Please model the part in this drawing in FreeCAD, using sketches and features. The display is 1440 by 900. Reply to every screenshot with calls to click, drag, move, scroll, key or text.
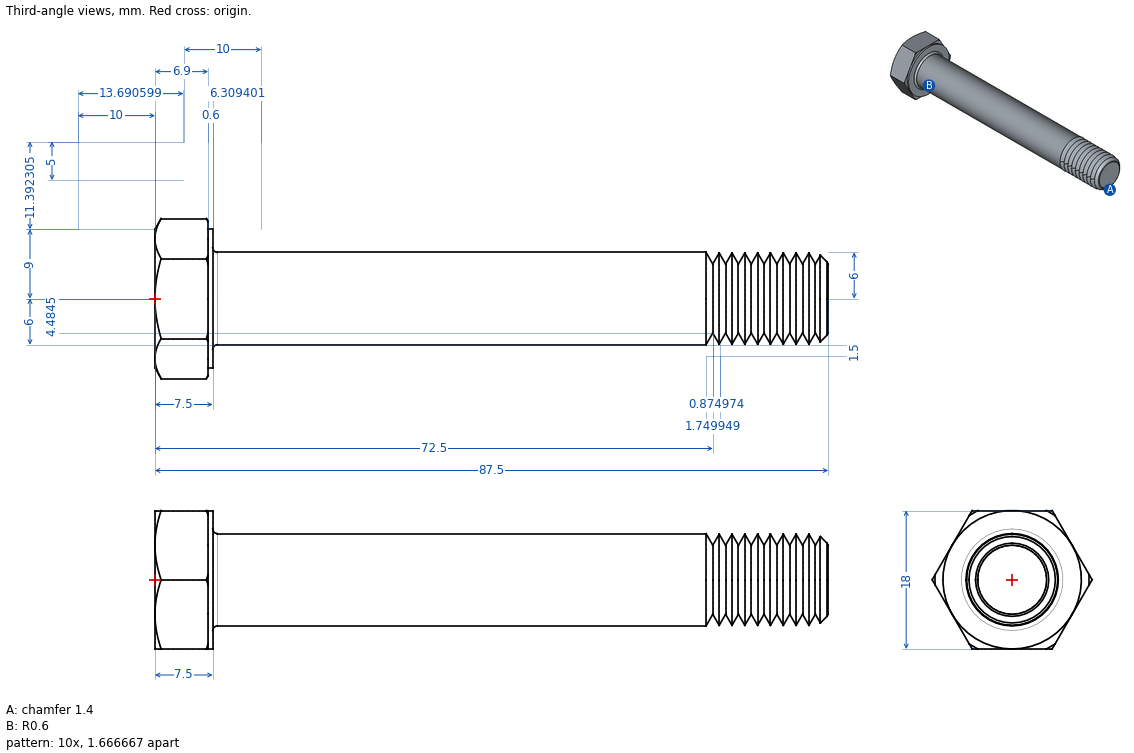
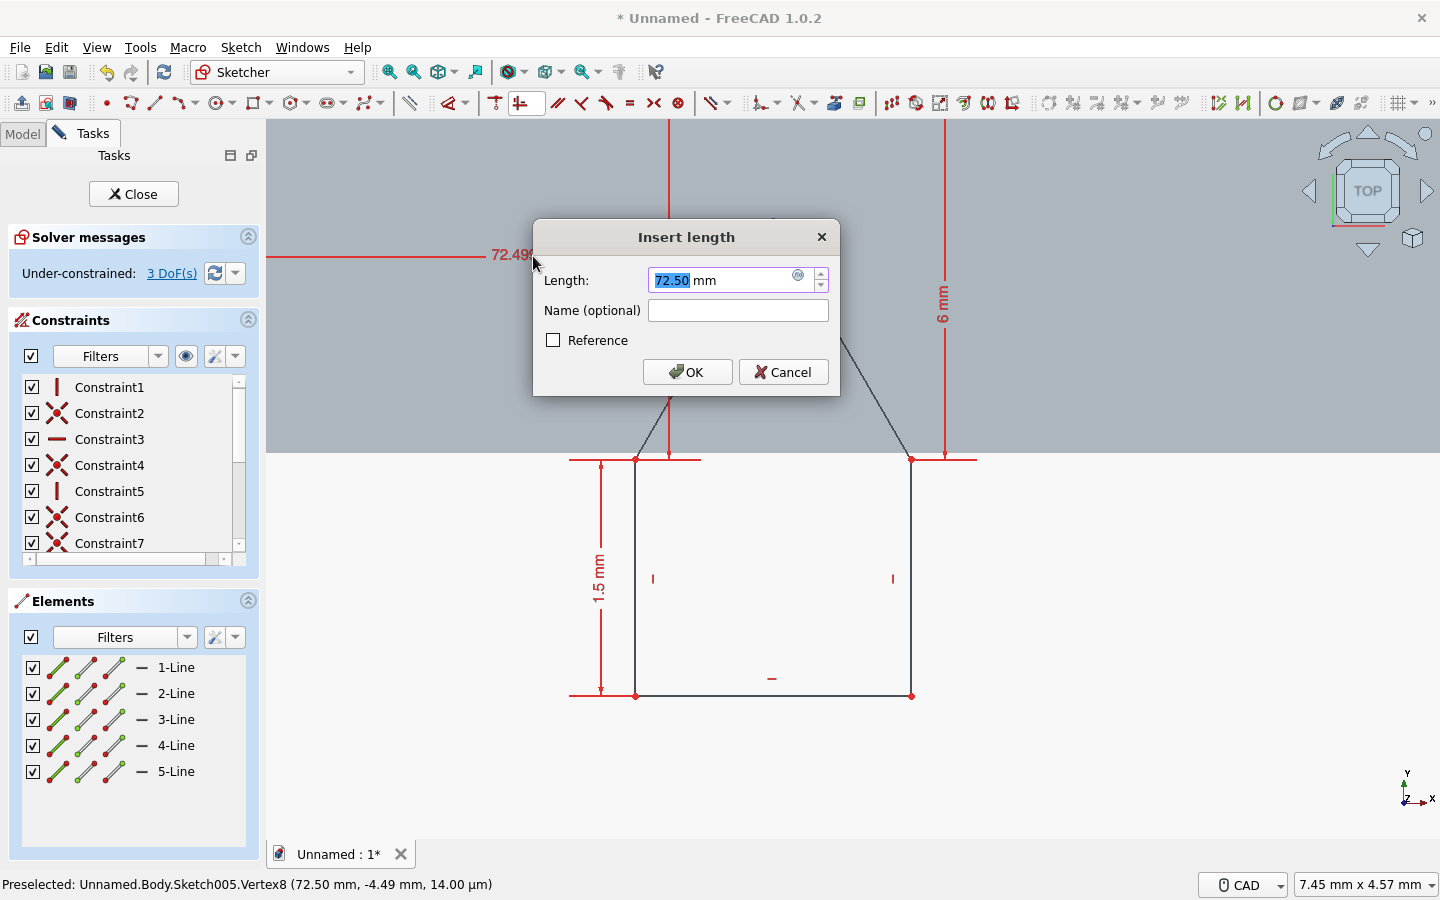
text(72.5)
key(Return)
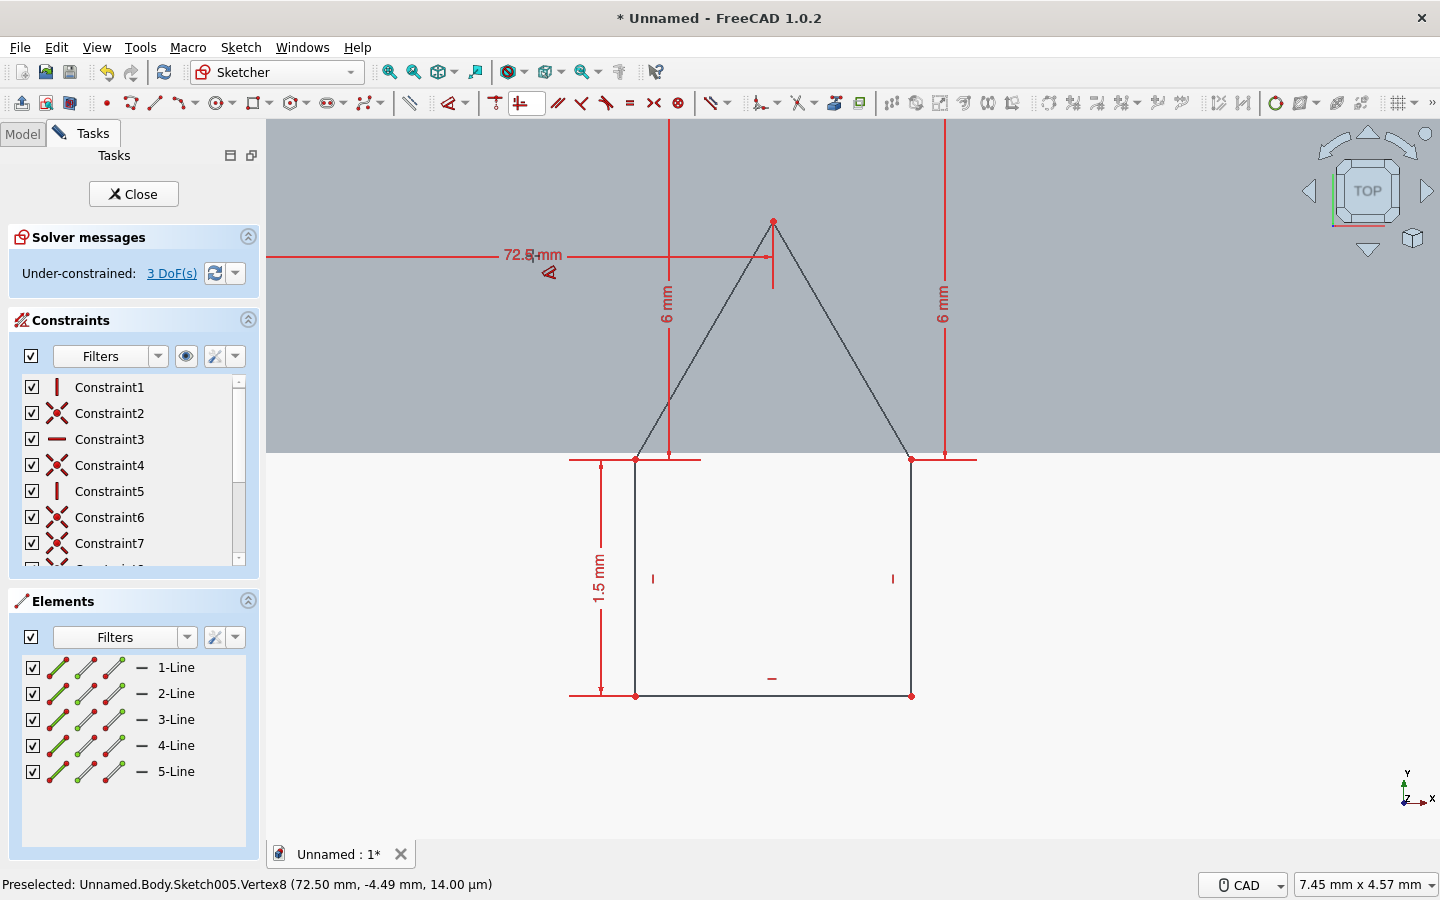
click(773, 222)
click(807, 184)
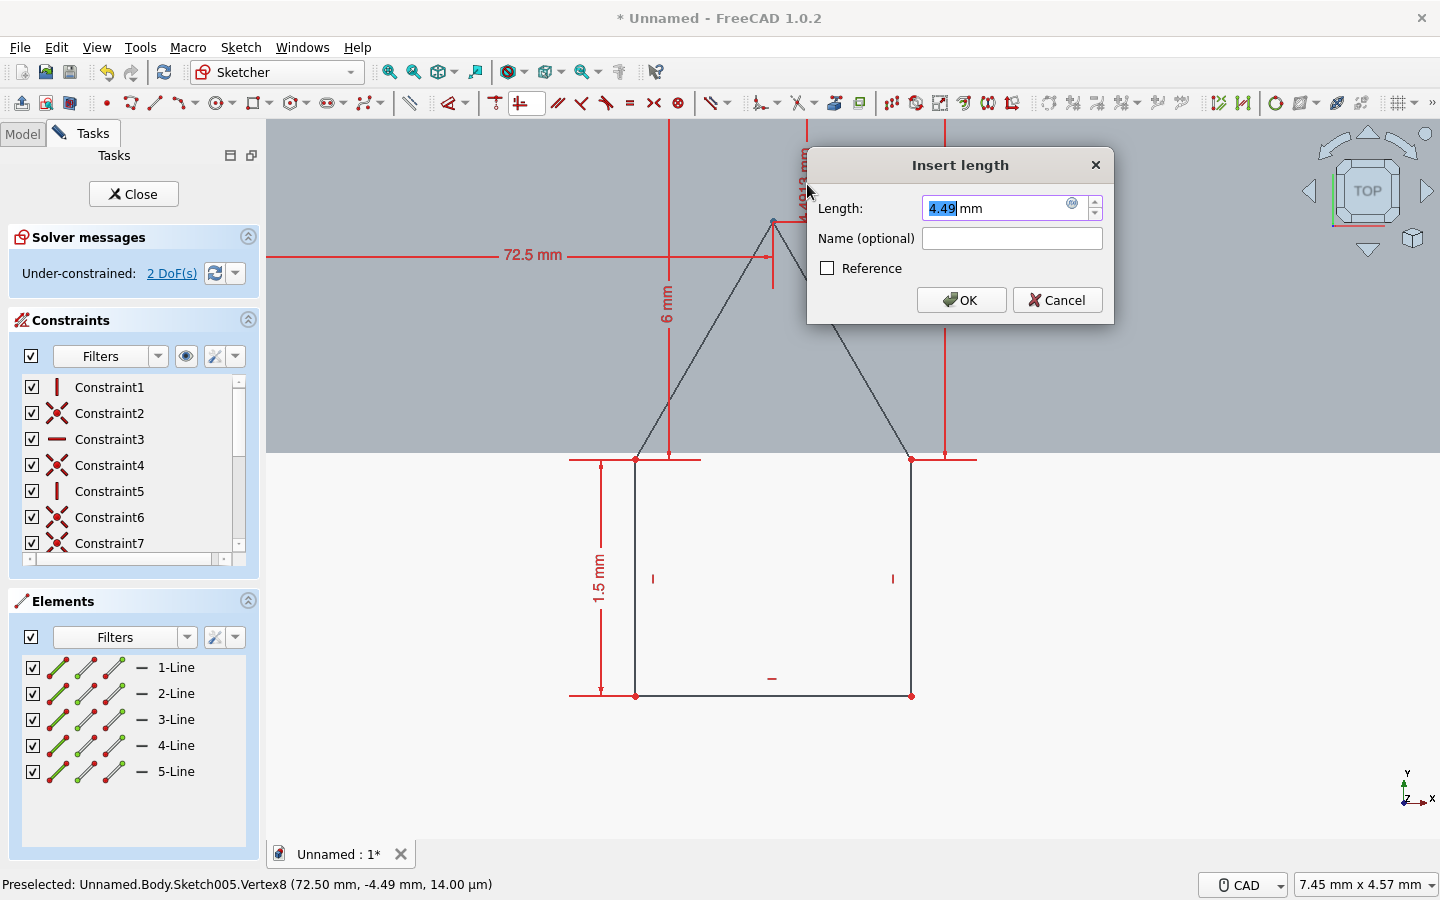
text(4.4845)
key(Return)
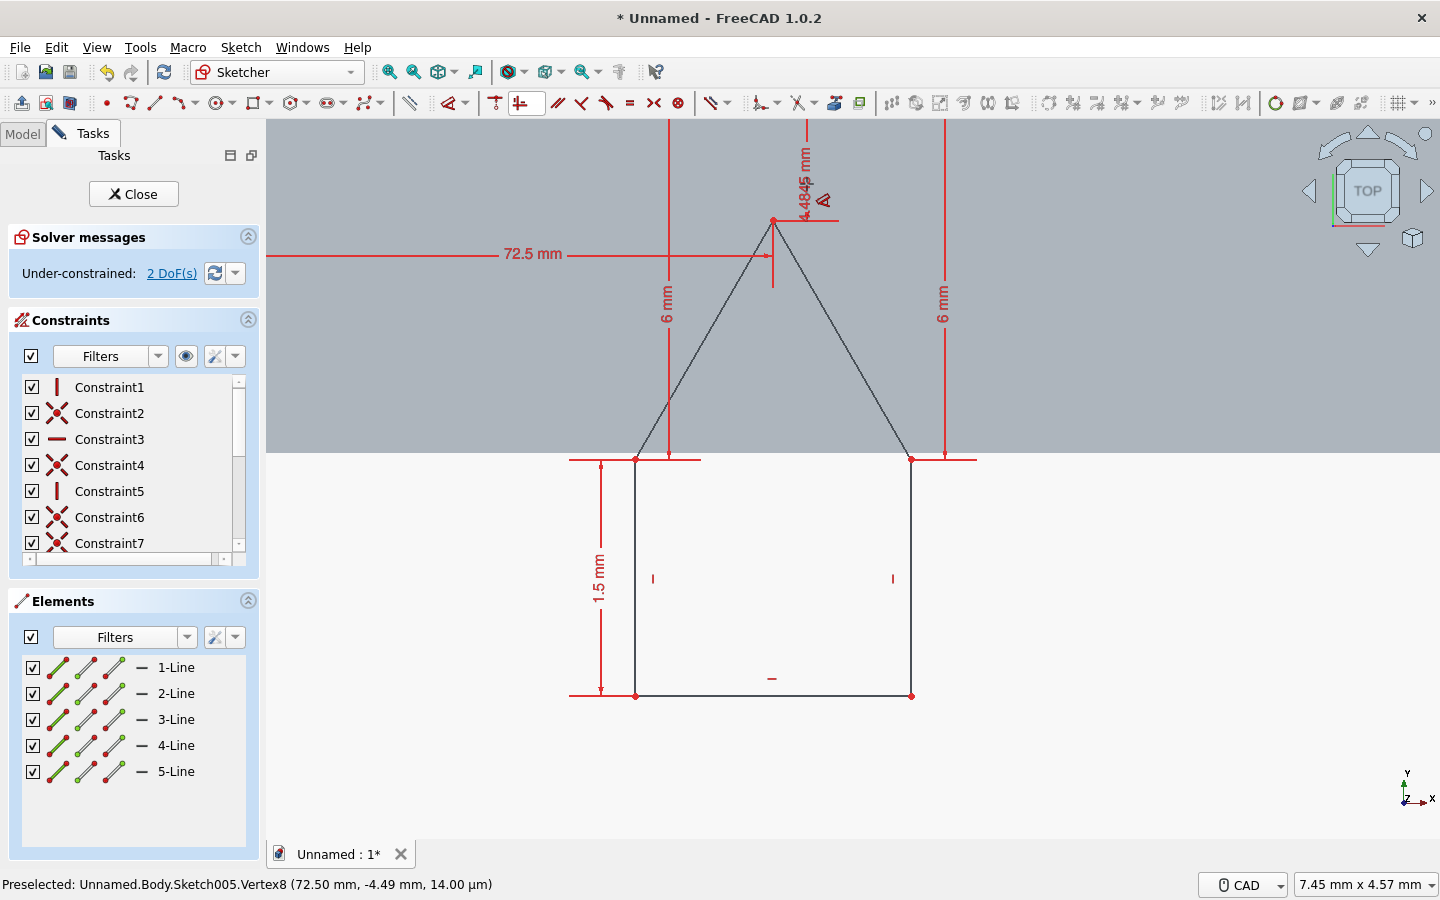
click(718, 696)
click(773, 730)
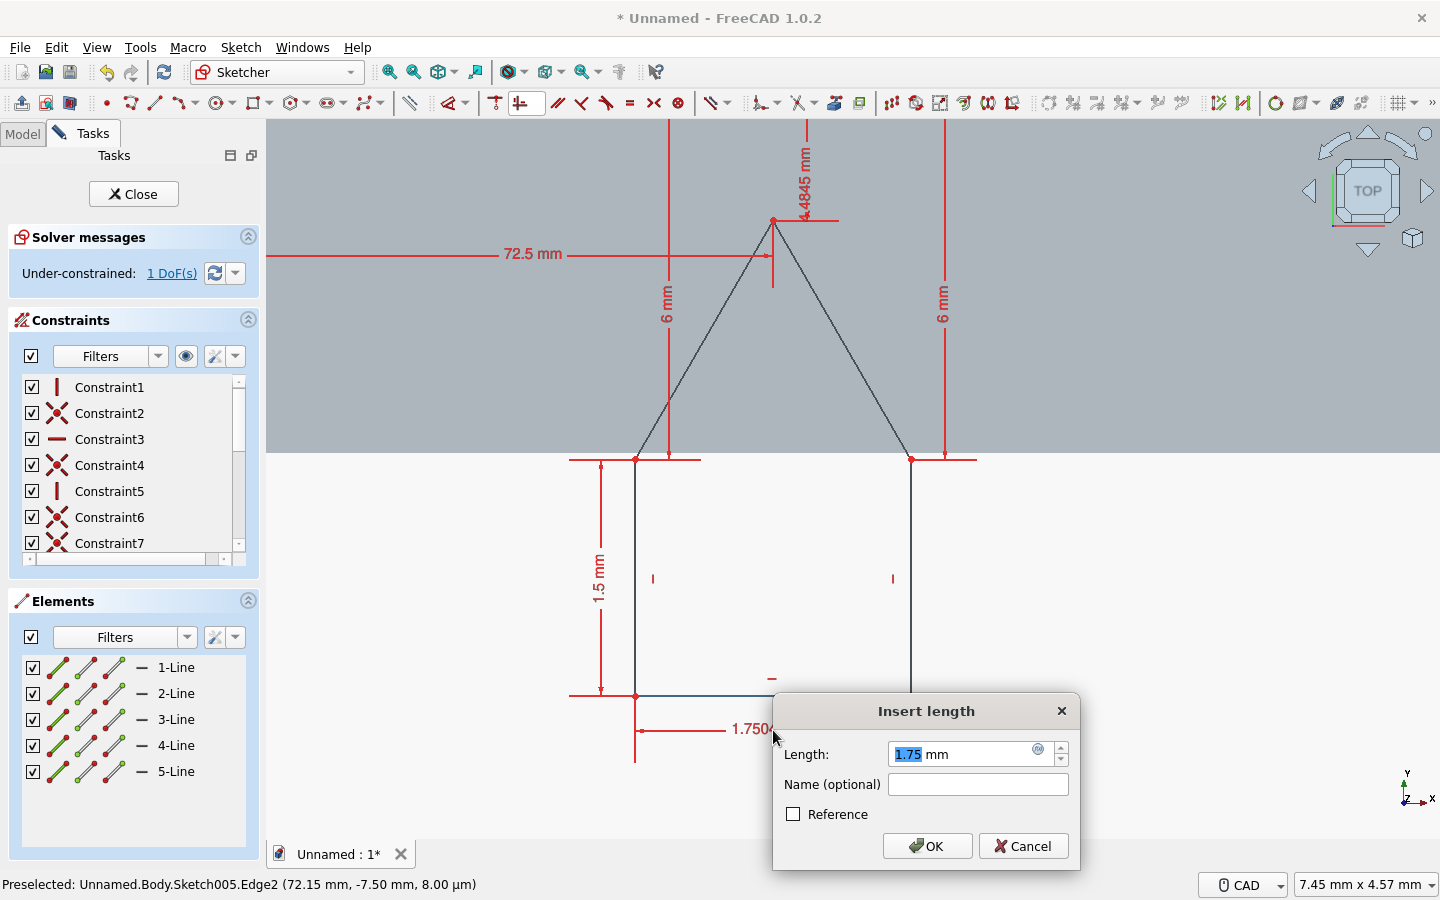
text(1.749949)
key(Return)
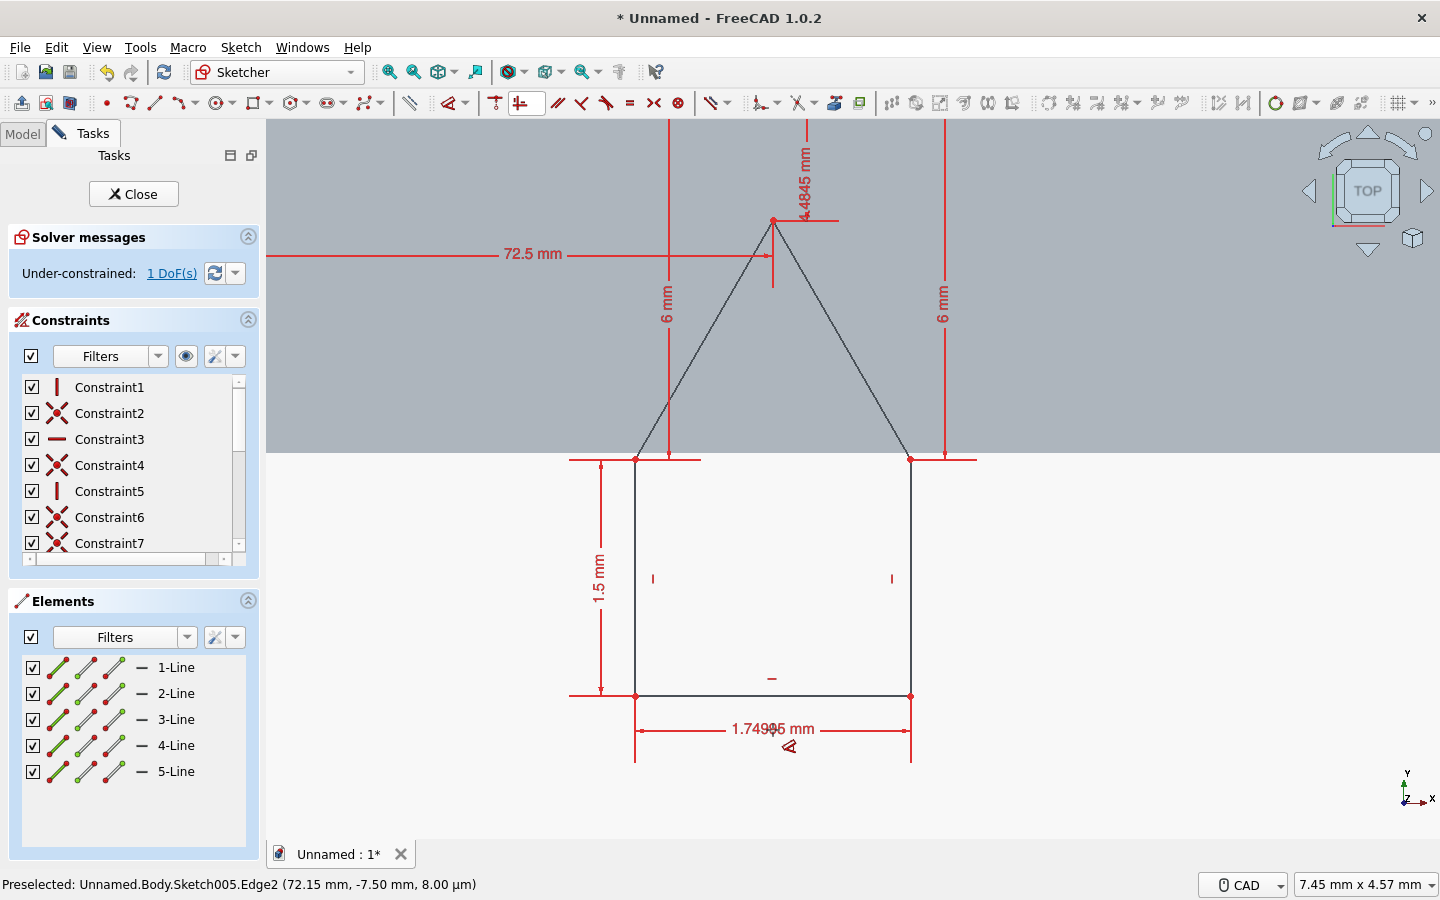
click(870, 388)
click(890, 187)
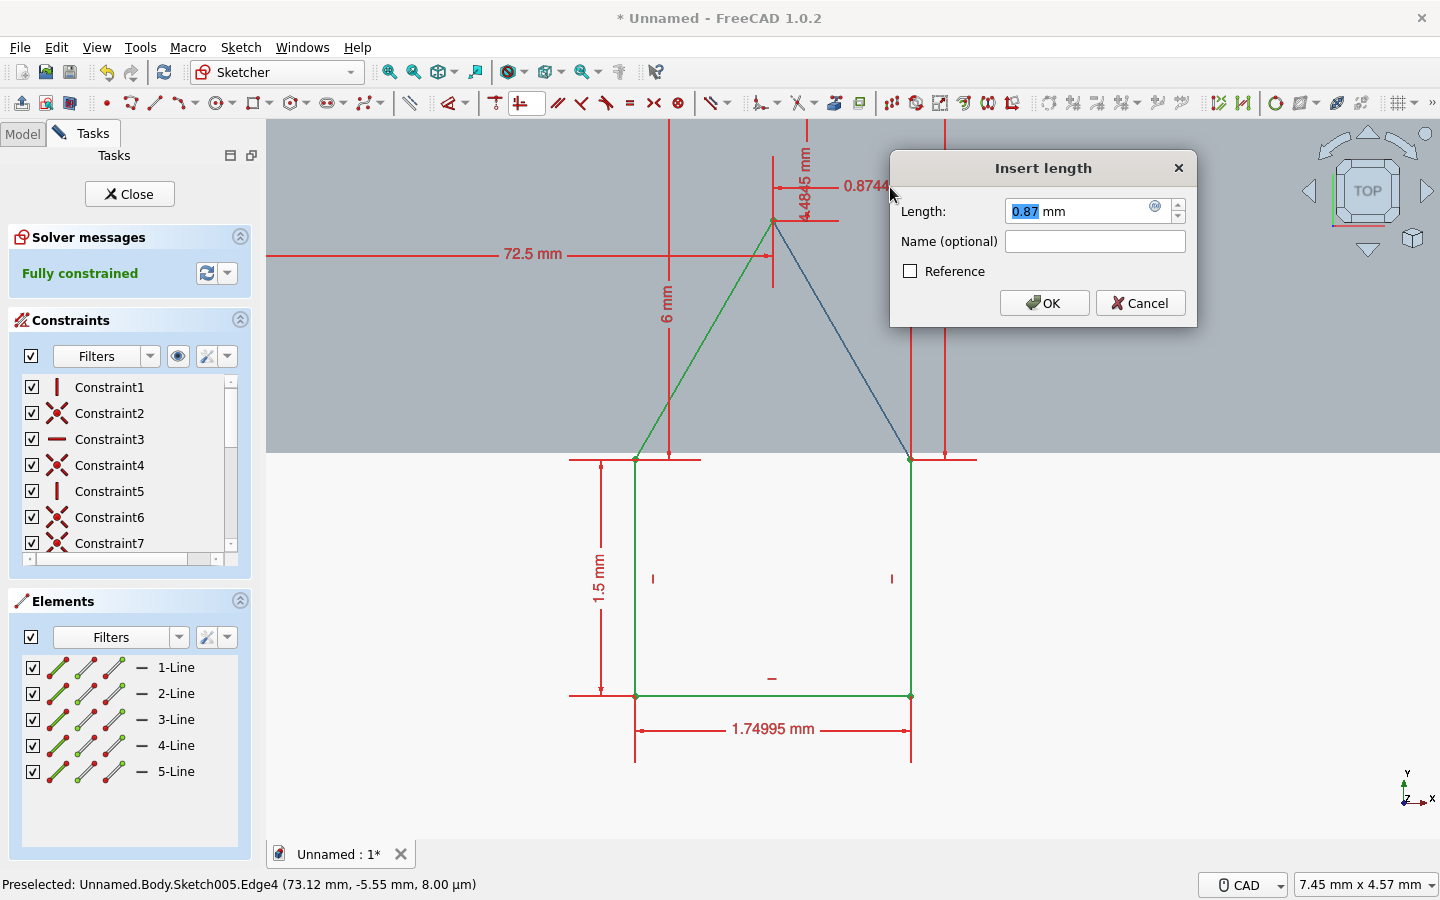
text(0.874974)
key(Return)
key(Escape)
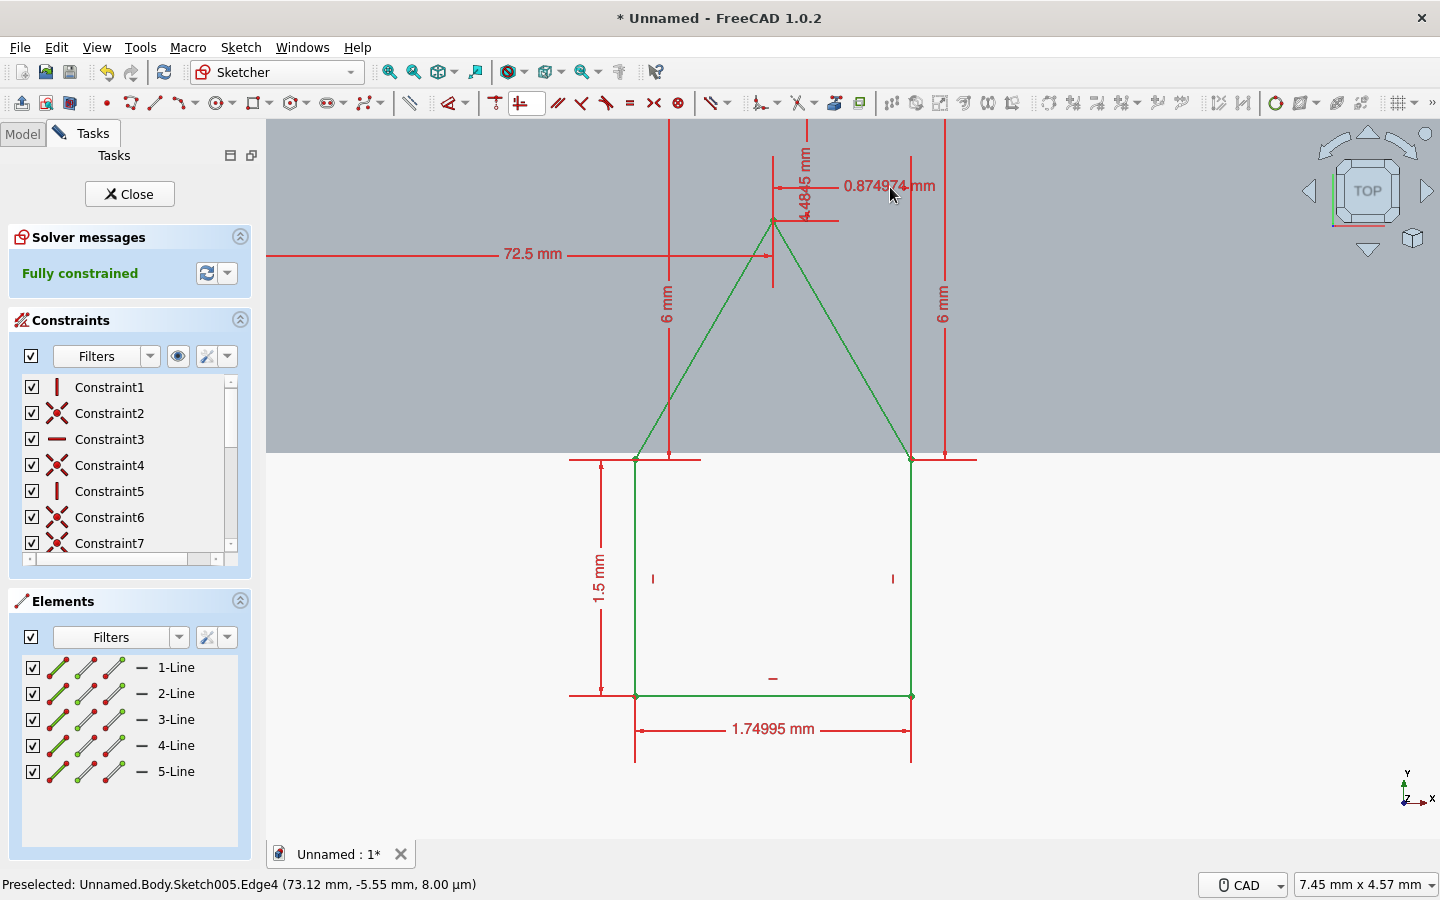
click(130, 194)